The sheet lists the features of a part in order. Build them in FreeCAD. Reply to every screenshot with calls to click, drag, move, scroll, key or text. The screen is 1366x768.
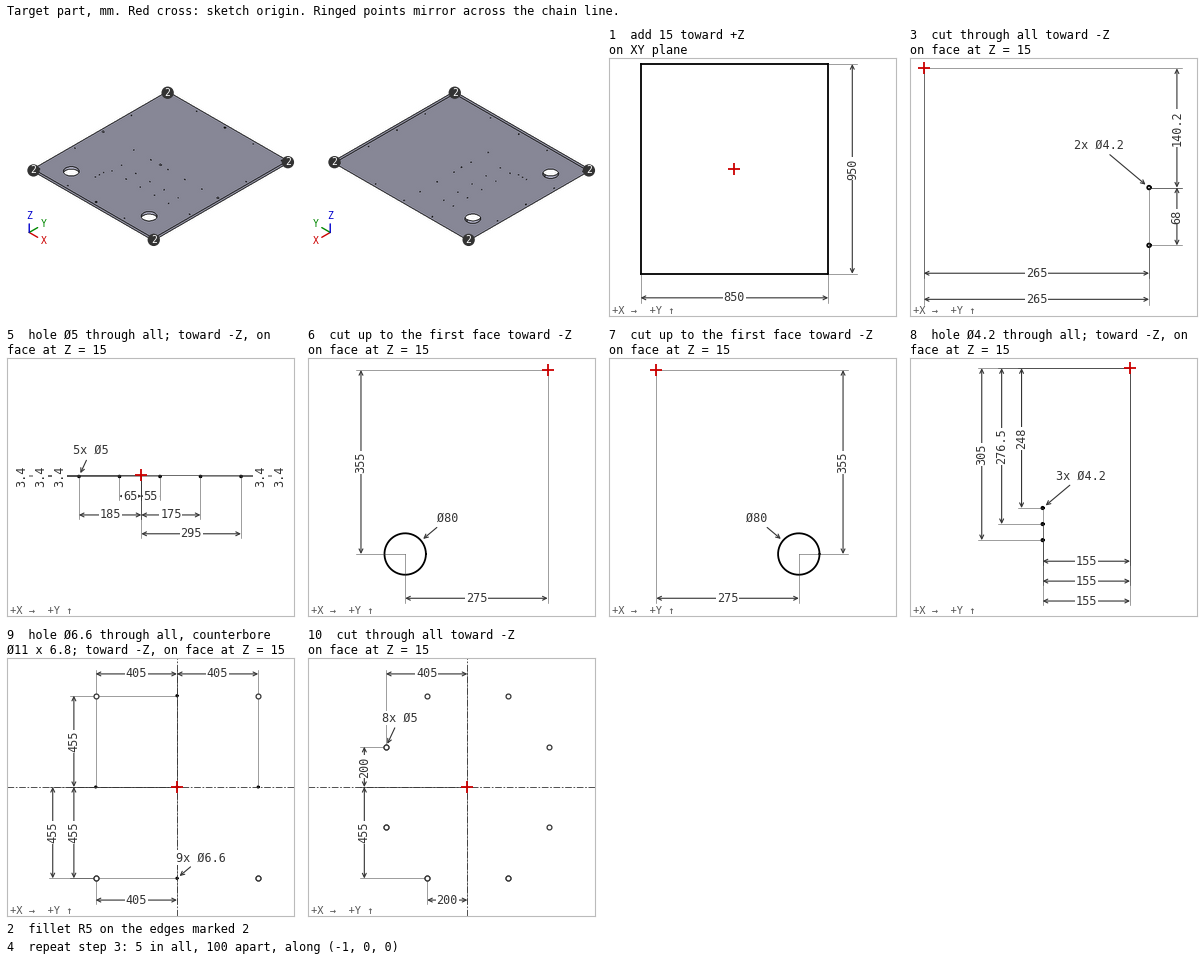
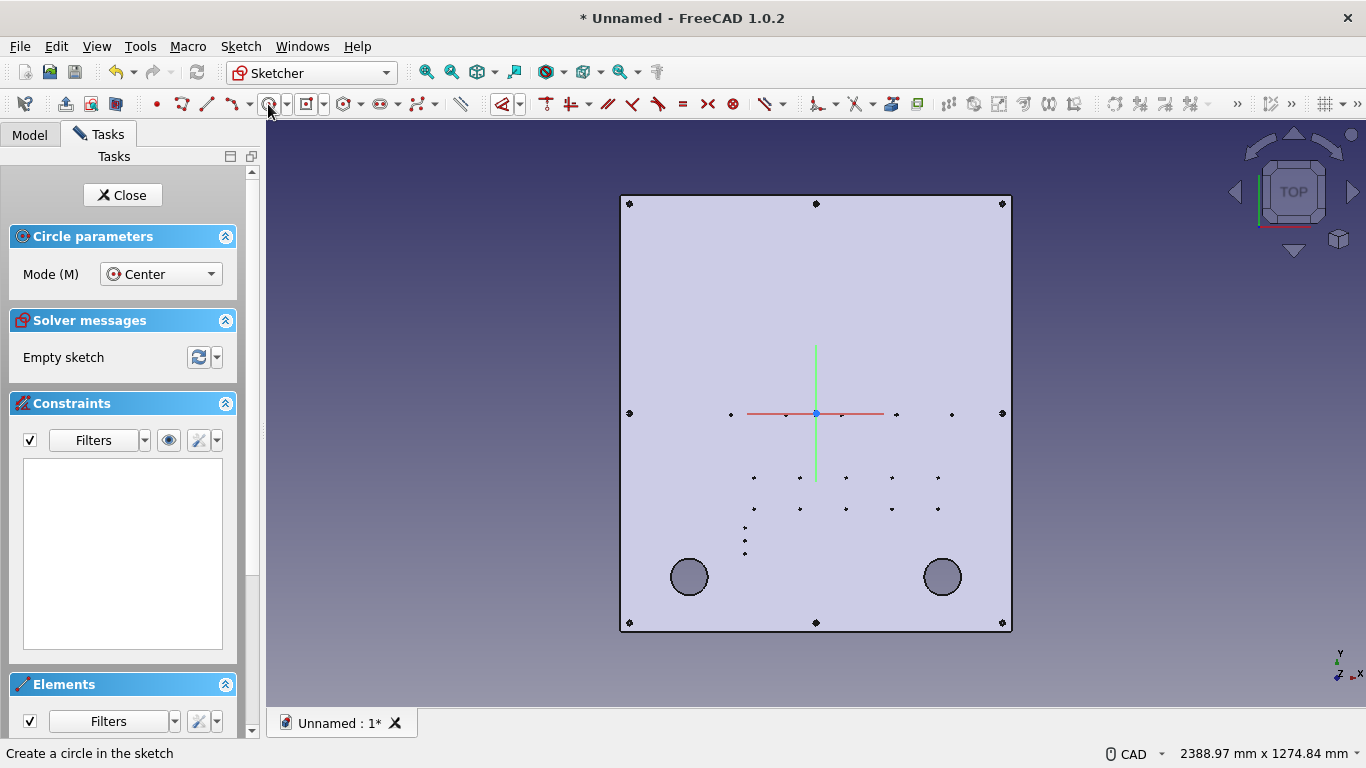
scroll(630, 321, up, 15)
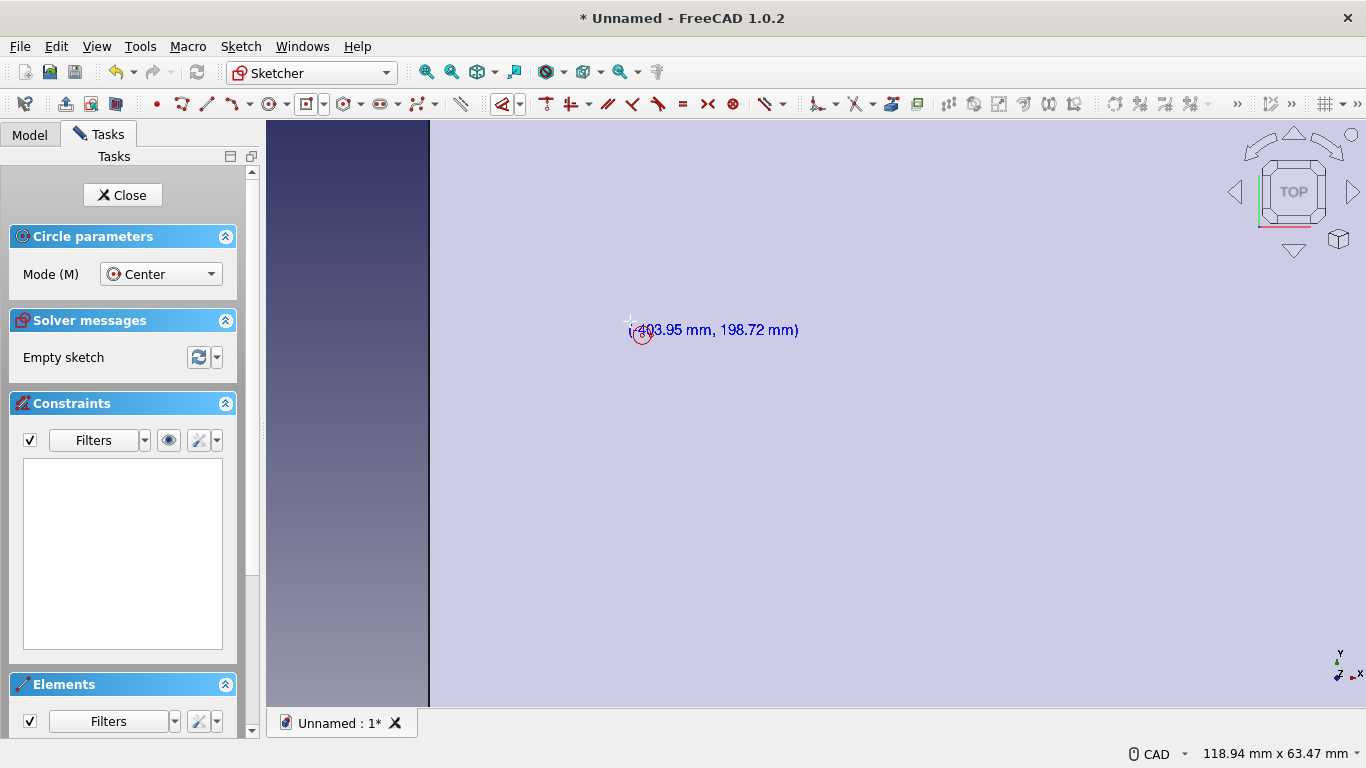
scroll(558, 321, down, 15)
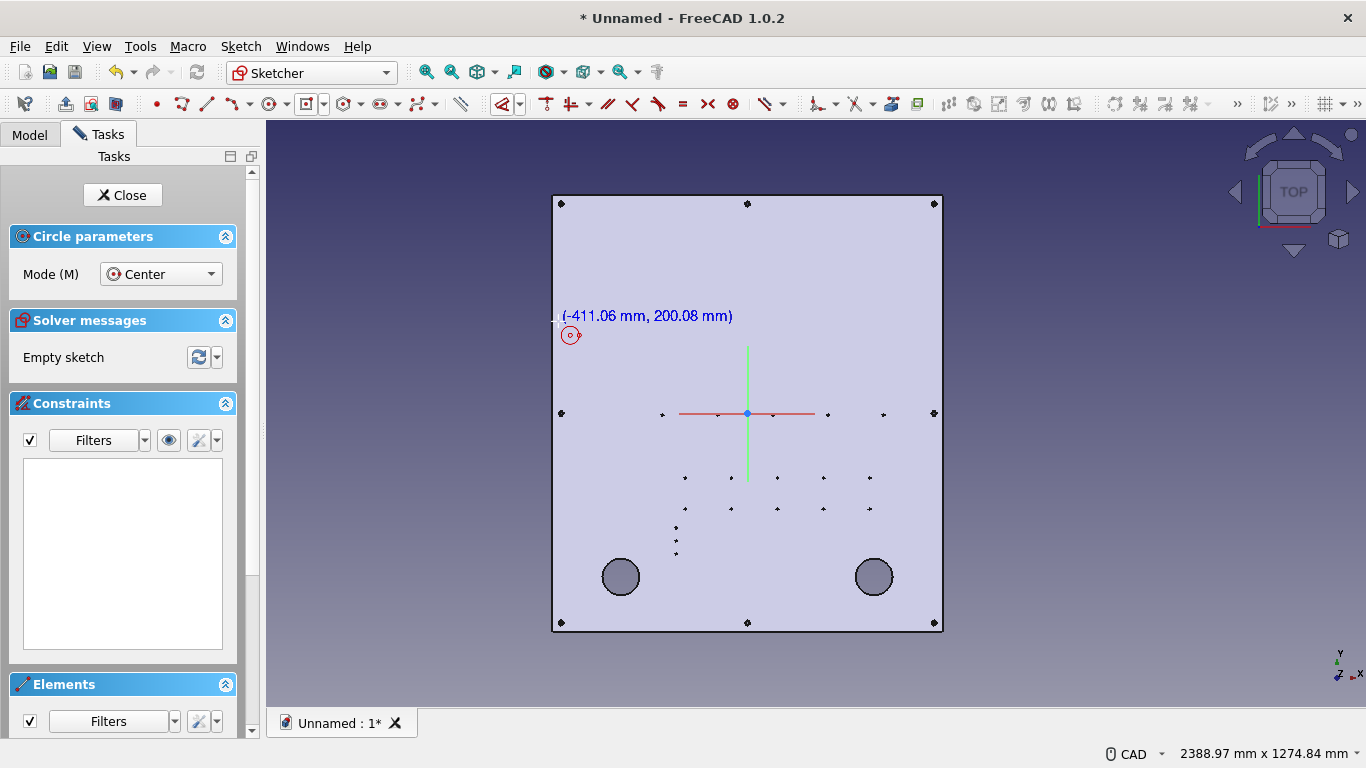
click(561, 321)
move(562, 321)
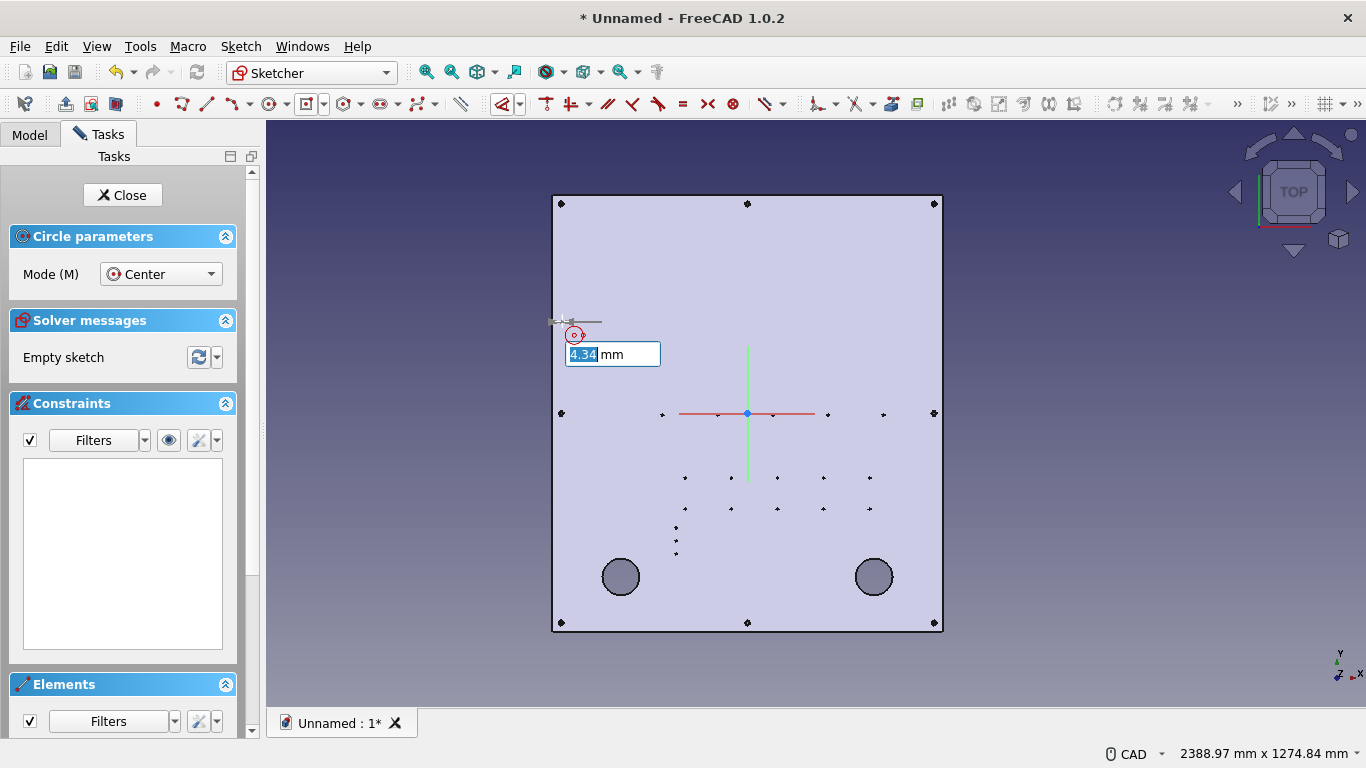
text(5)
key(Return)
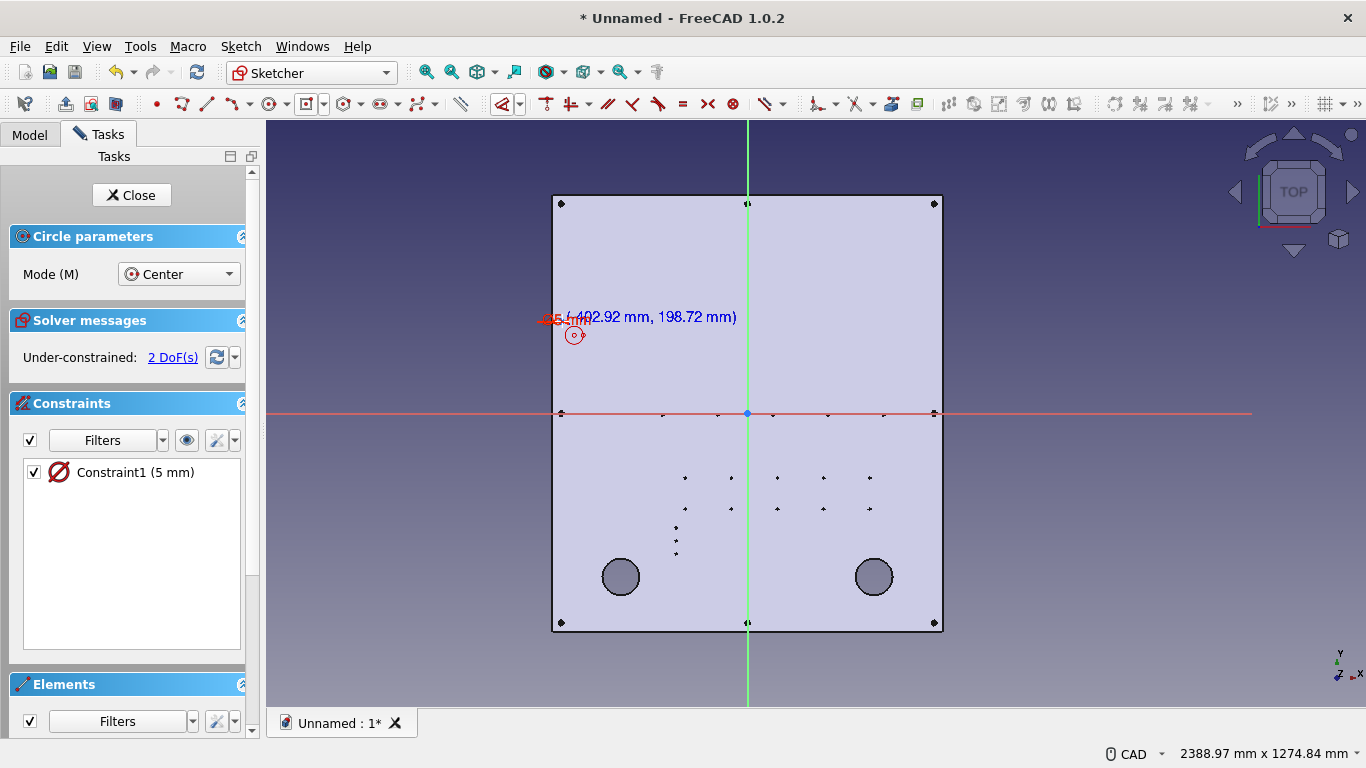
scroll(561, 506, up, 15)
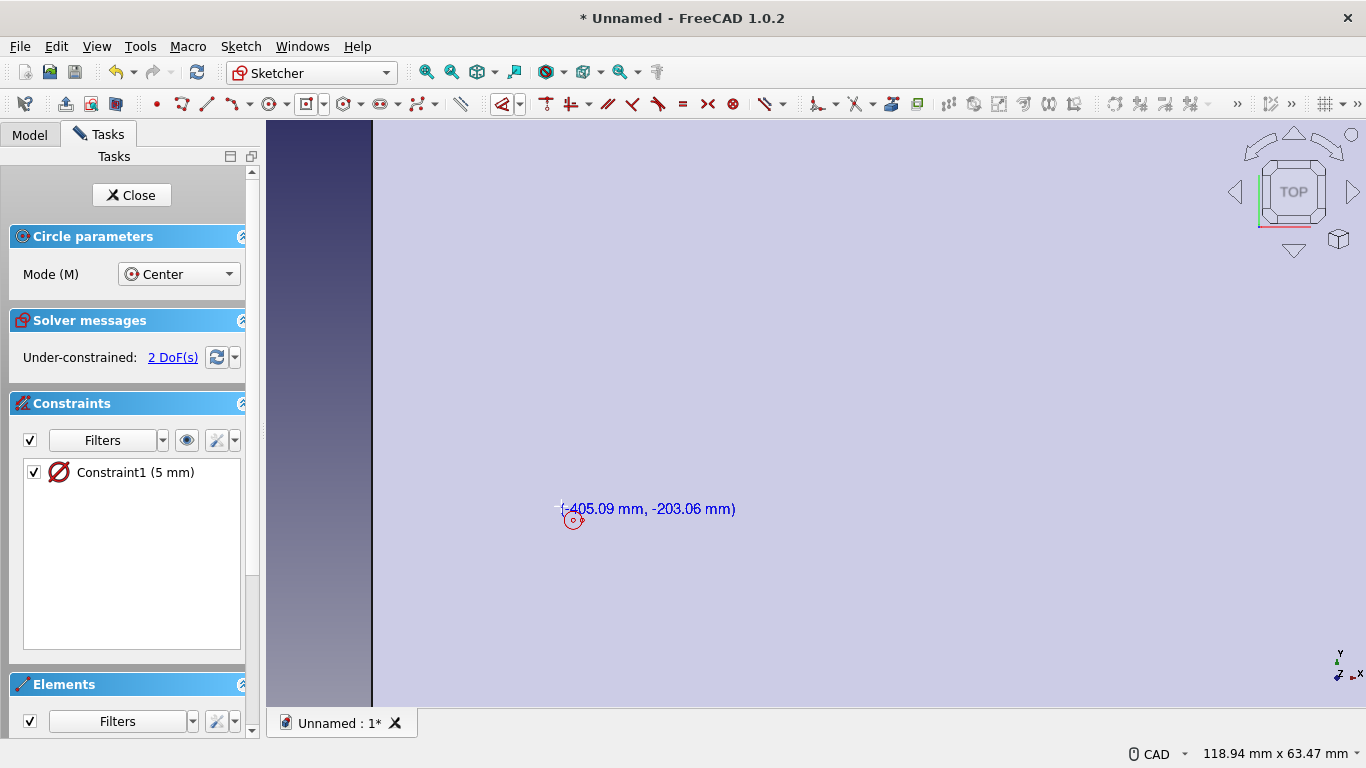
scroll(561, 507, down, 15)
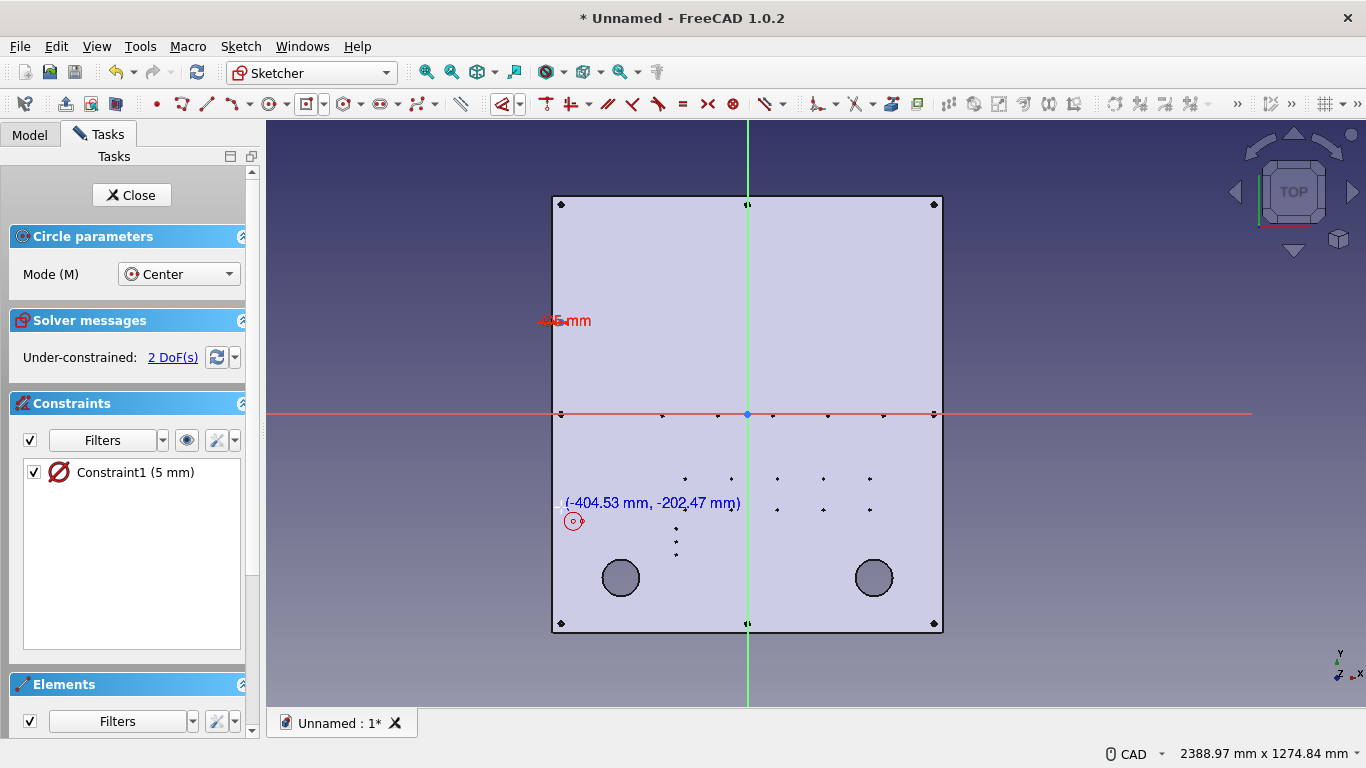
click(561, 507)
move(562, 506)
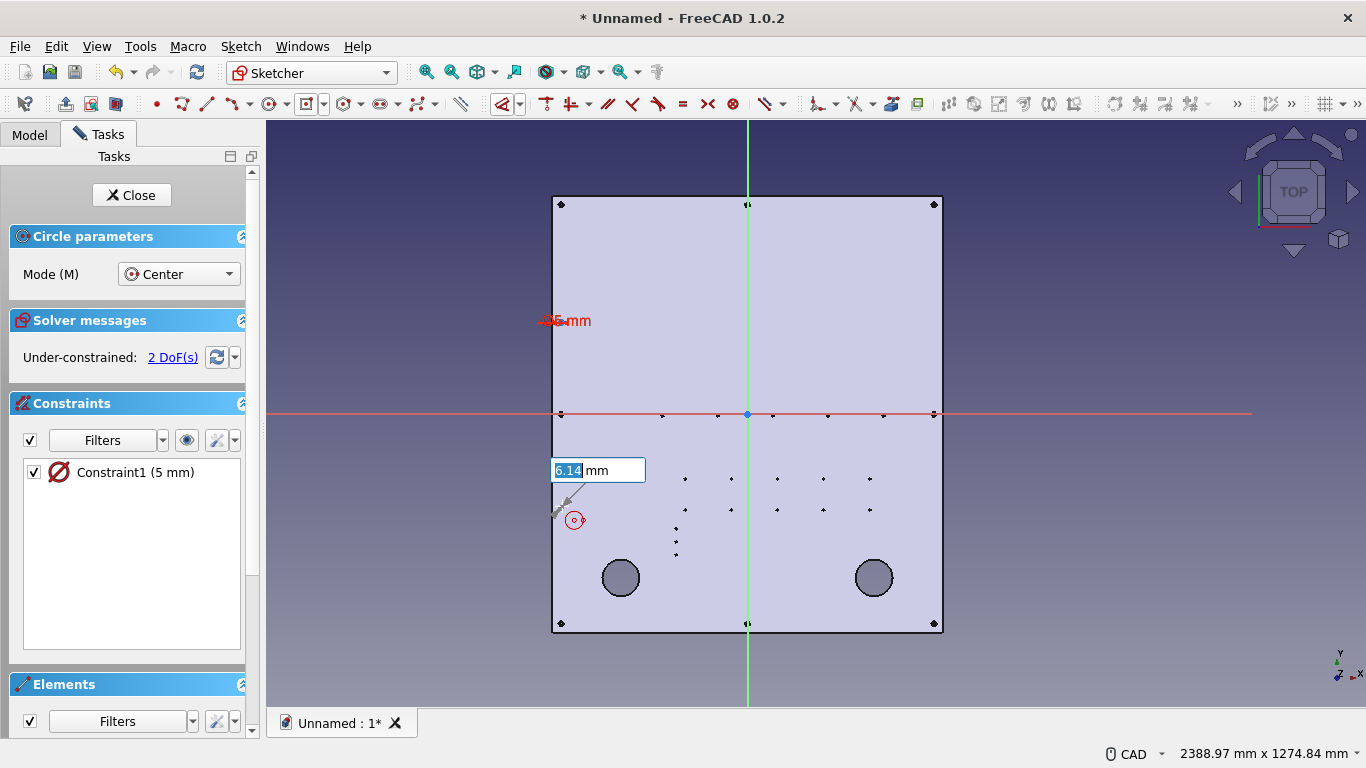
text(5)
key(Return)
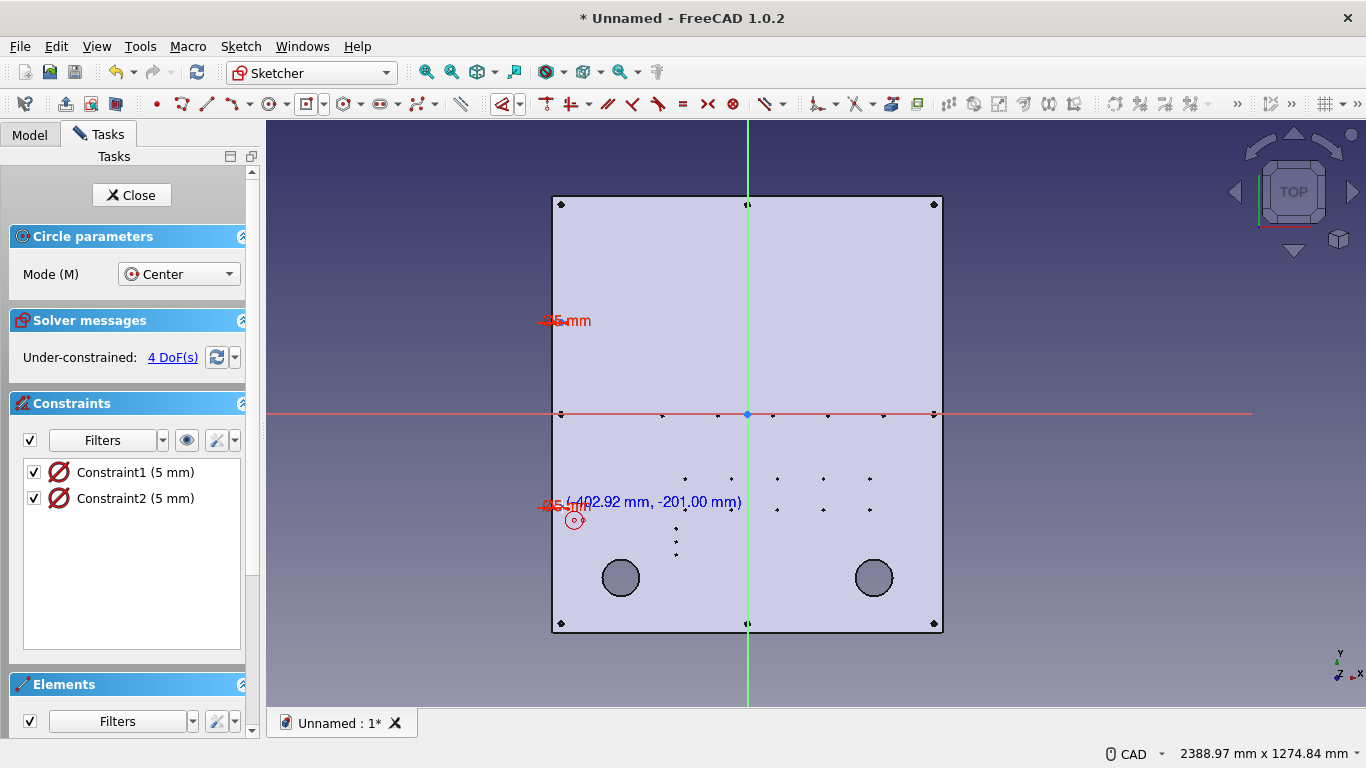
scroll(655, 624, up, 15)